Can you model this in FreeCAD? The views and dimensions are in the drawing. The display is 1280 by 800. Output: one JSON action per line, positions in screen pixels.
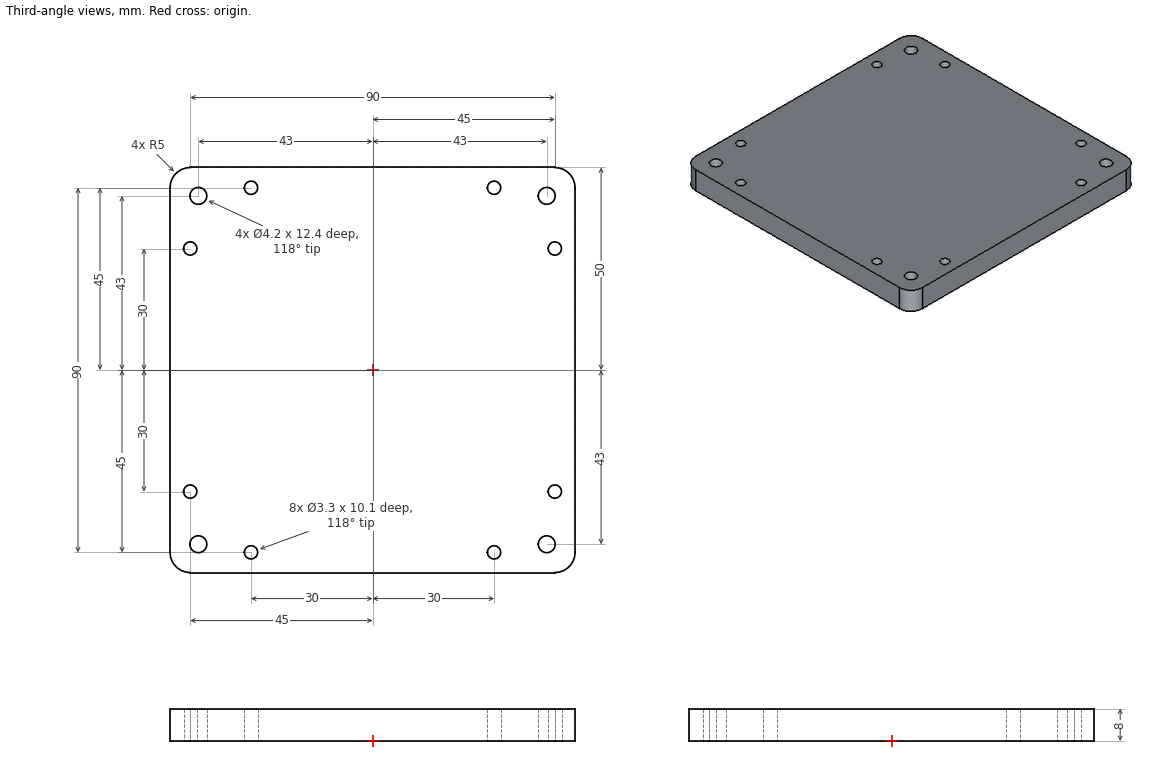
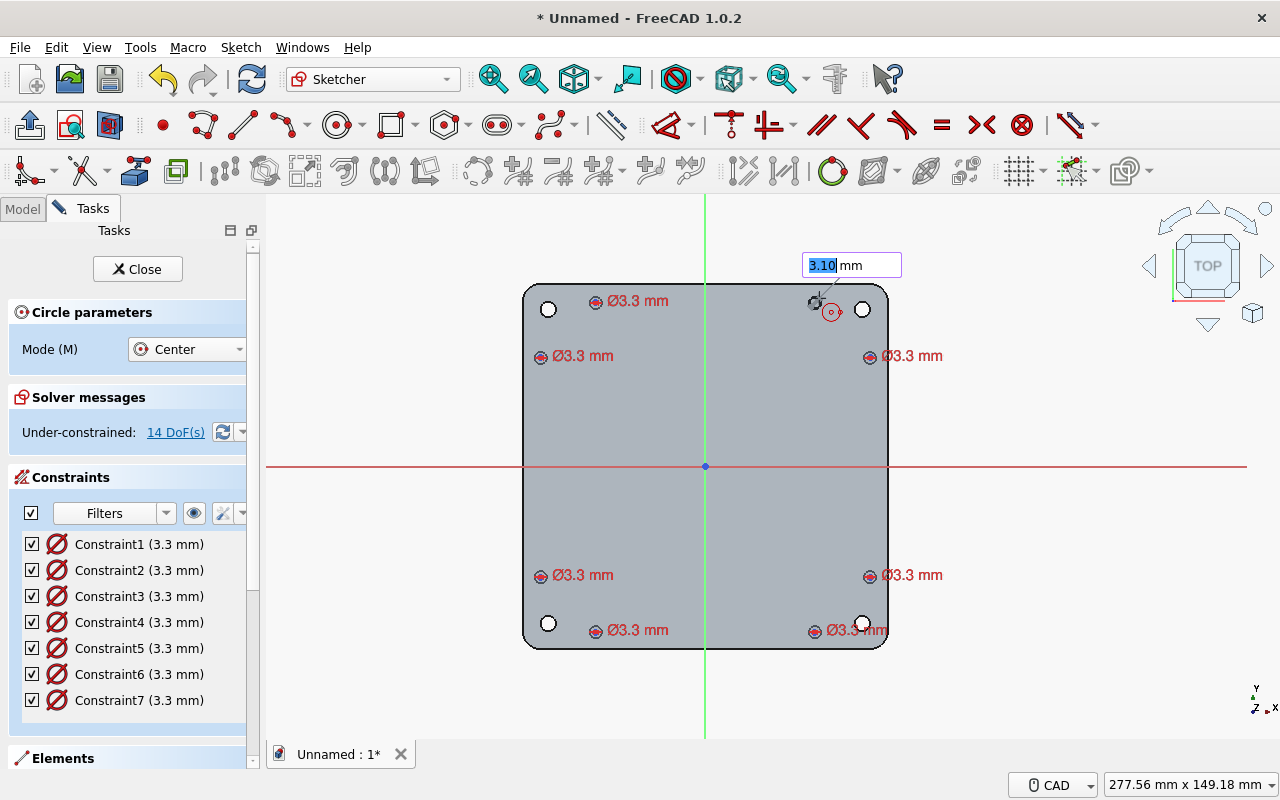
{"action": "type", "text": "3.3"}
{"action": "key", "text": "Return"}
{"action": "key", "text": "Escape"}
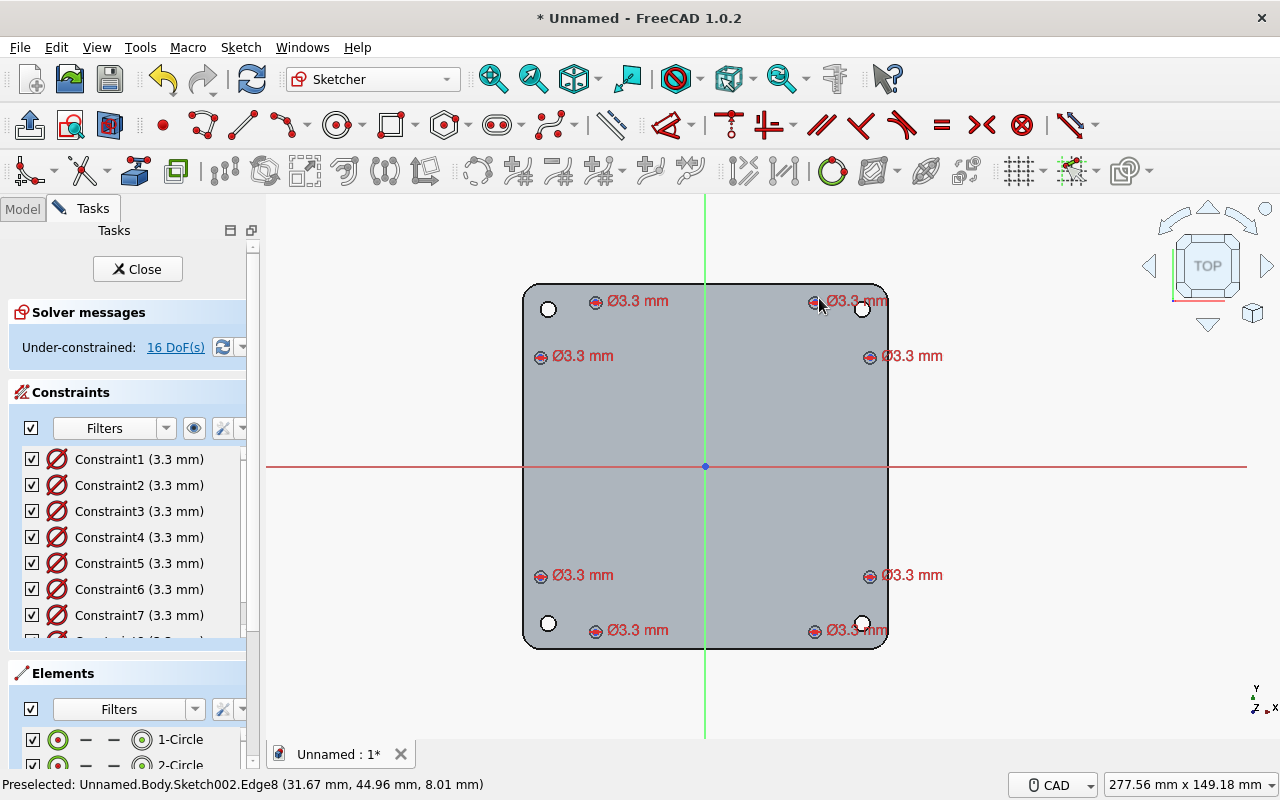
{"action": "left_click", "coordinate": [596, 632]}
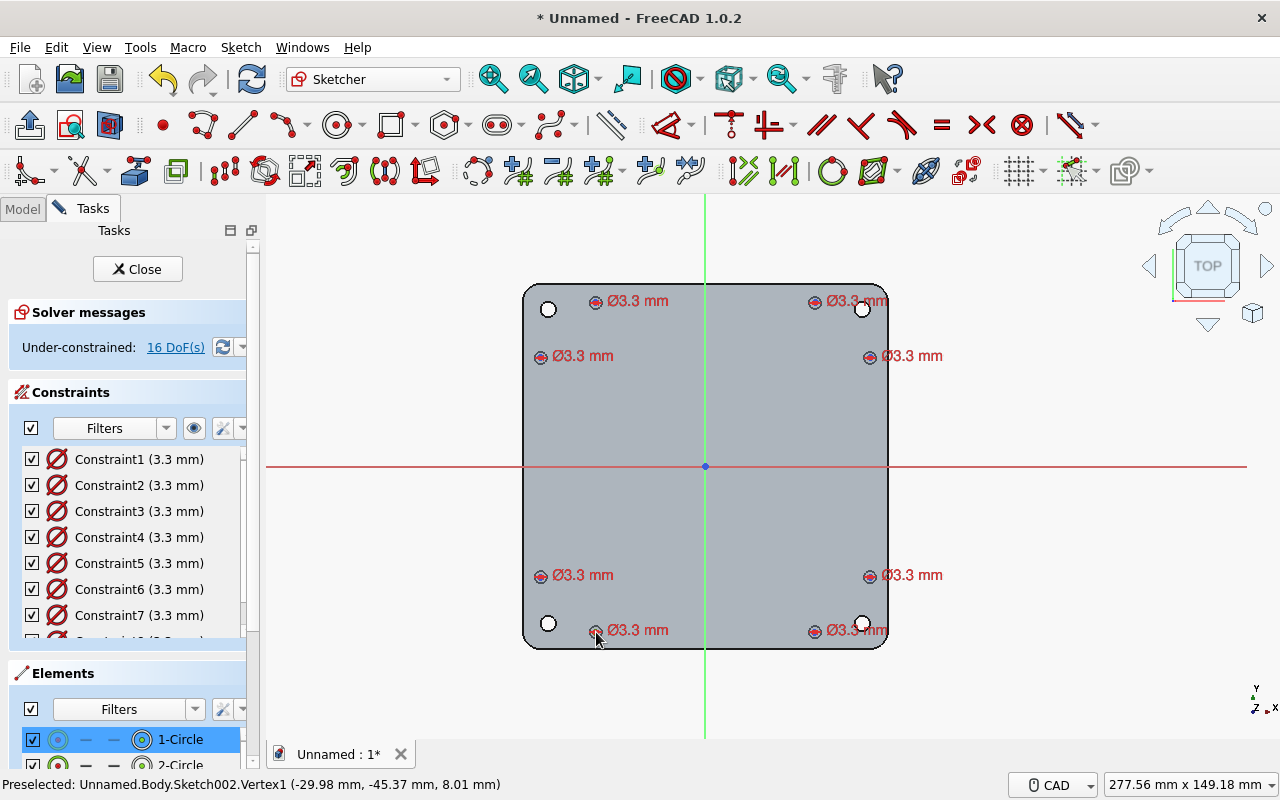
{"action": "left_click", "coordinate": [815, 632]}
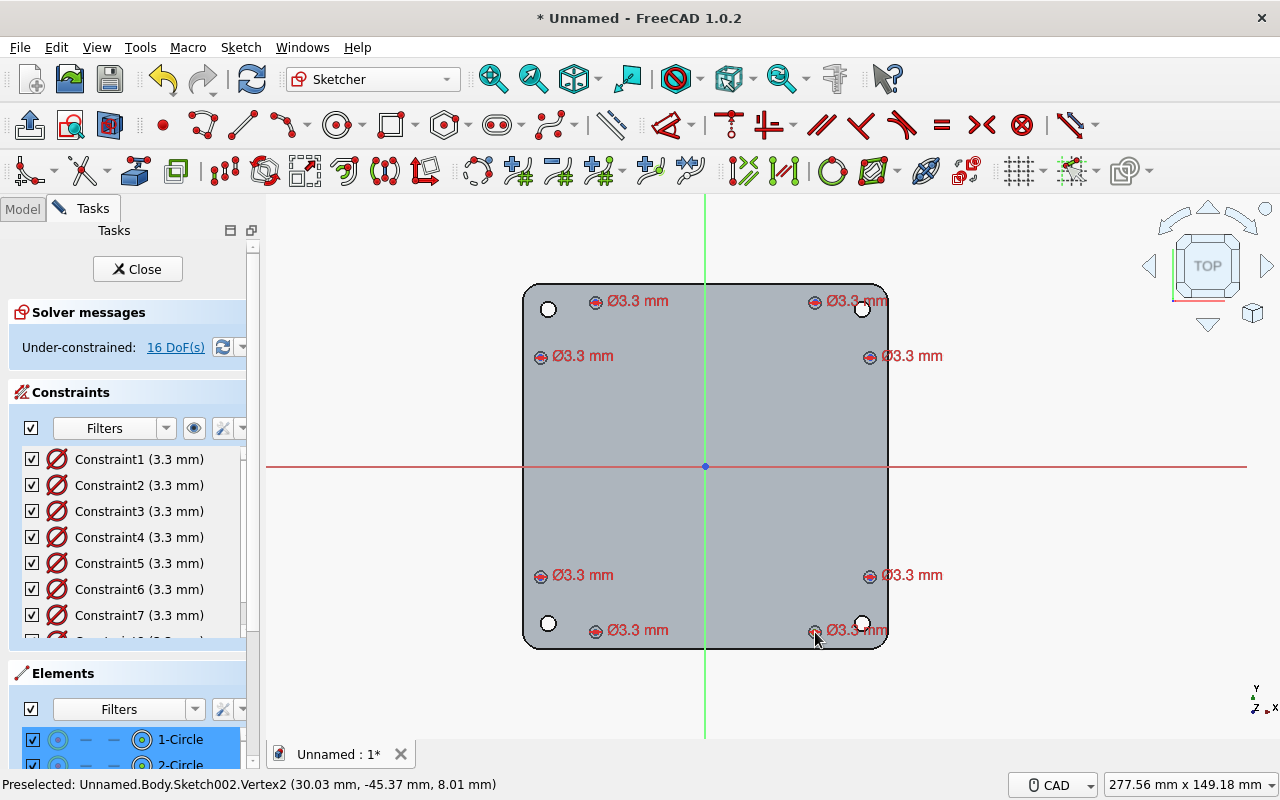
{"action": "key", "text": "h"}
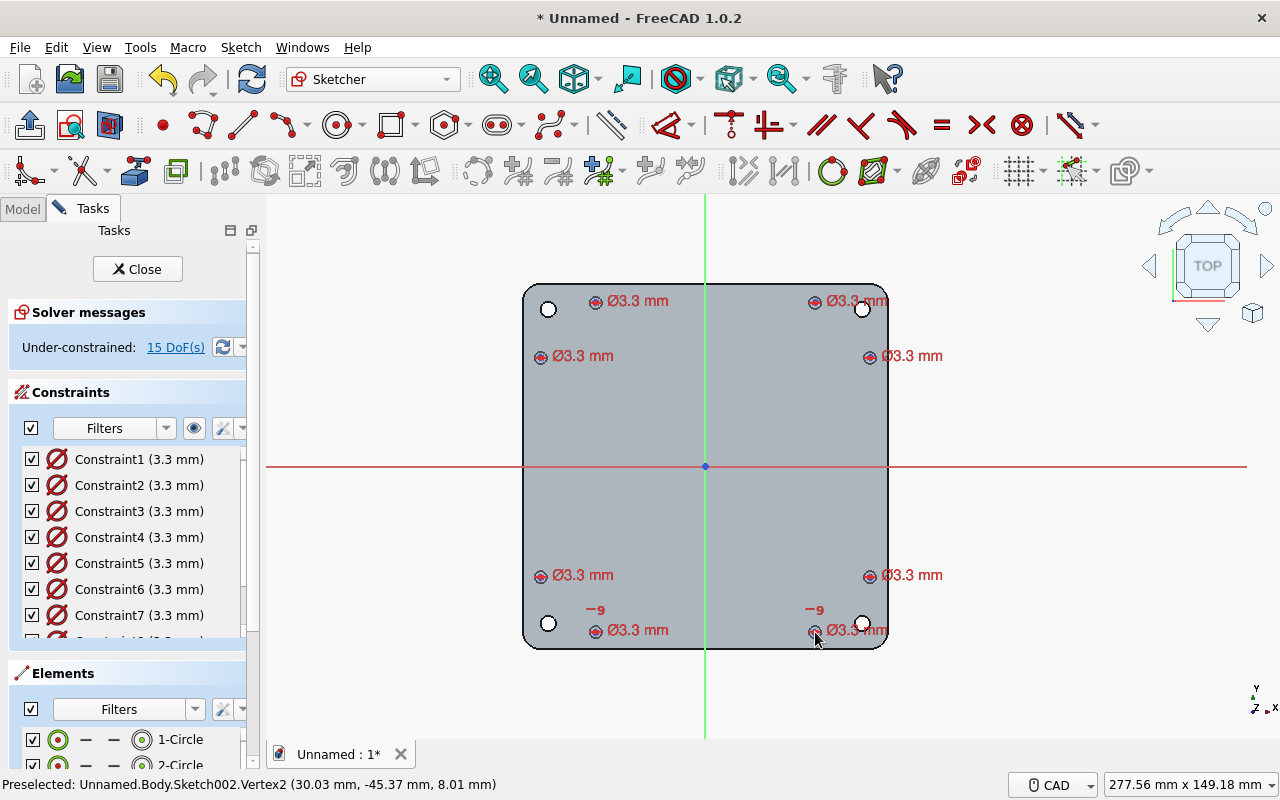
{"action": "left_click", "coordinate": [541, 577]}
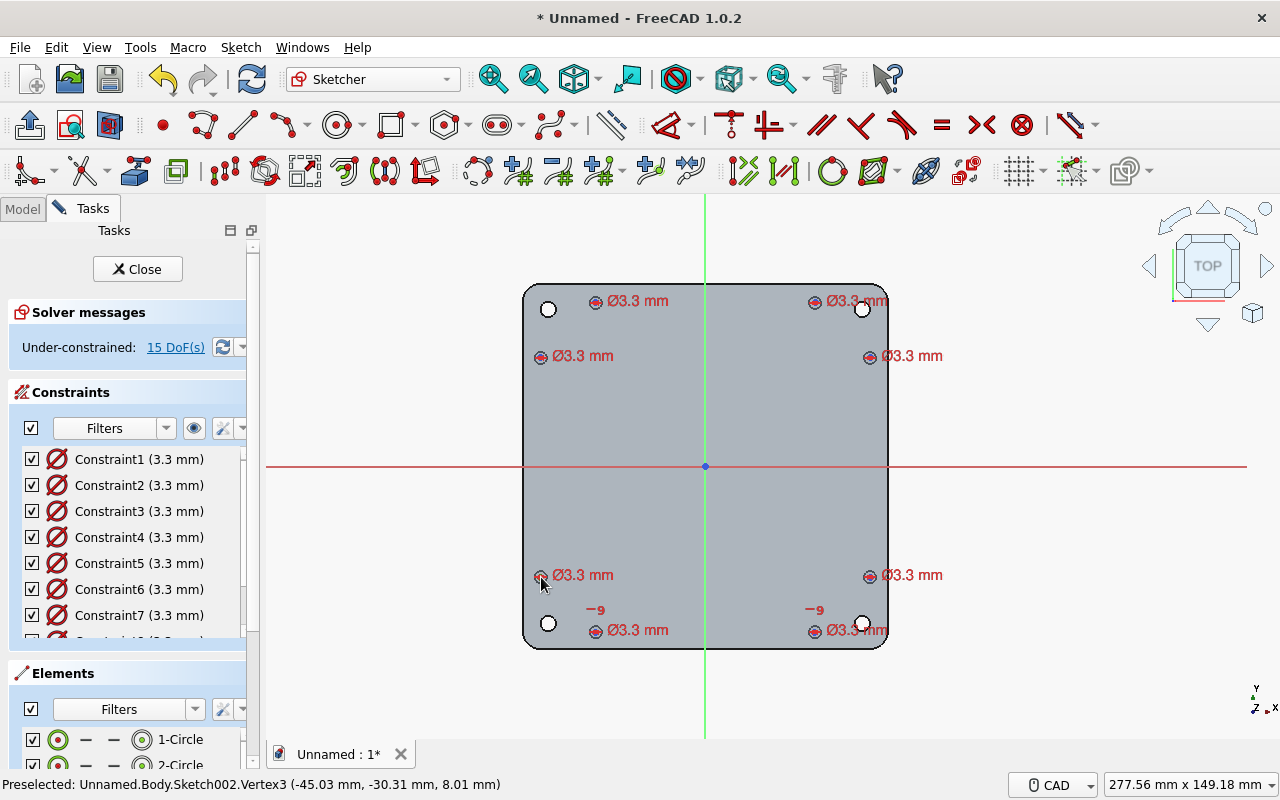
{"action": "left_click", "coordinate": [541, 358]}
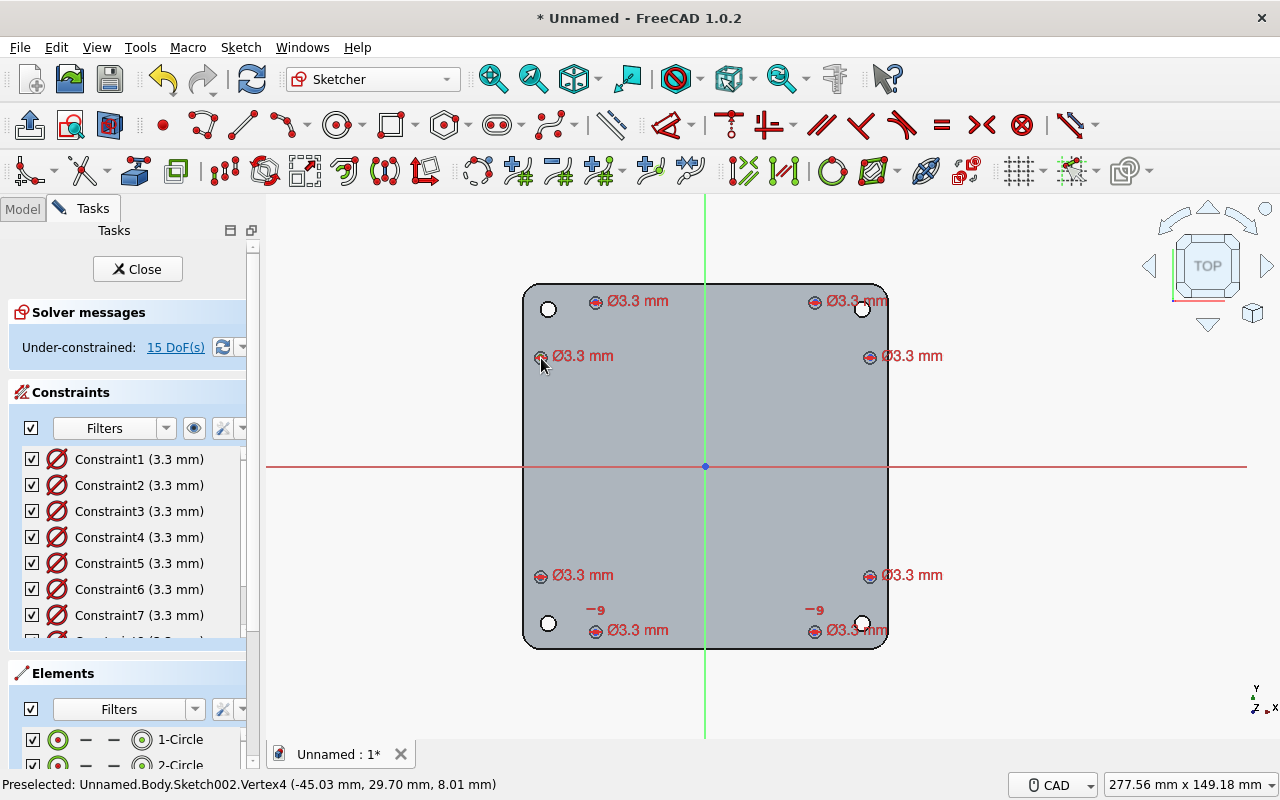
{"action": "key", "text": "v"}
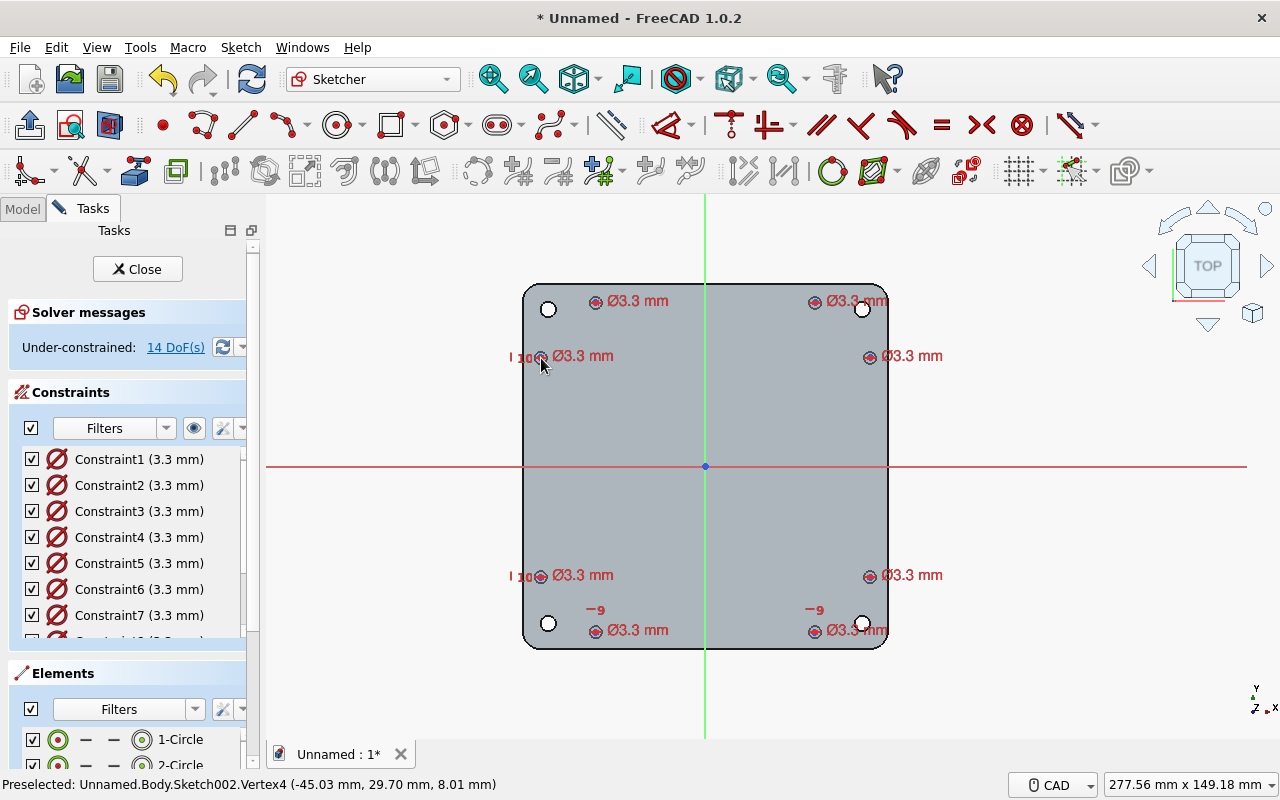
{"action": "left_click", "coordinate": [541, 358]}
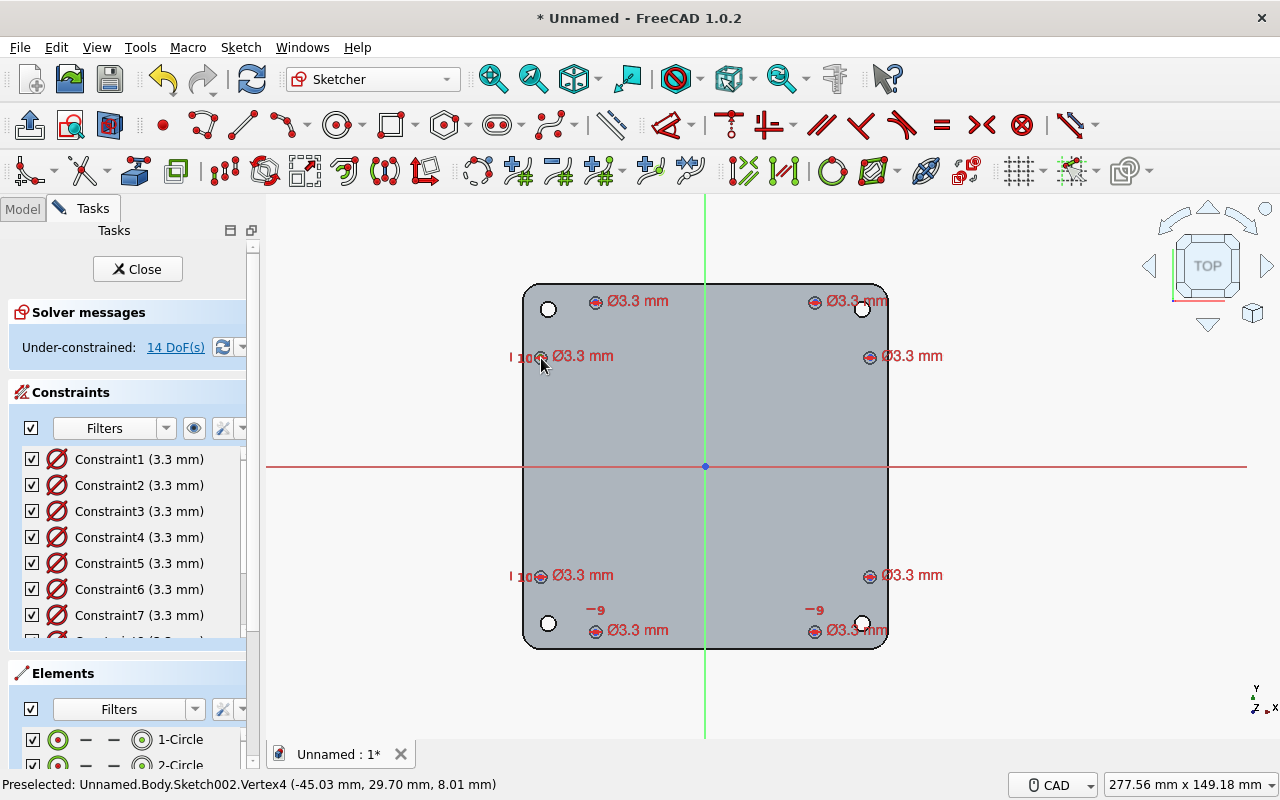
{"action": "left_click", "coordinate": [870, 358]}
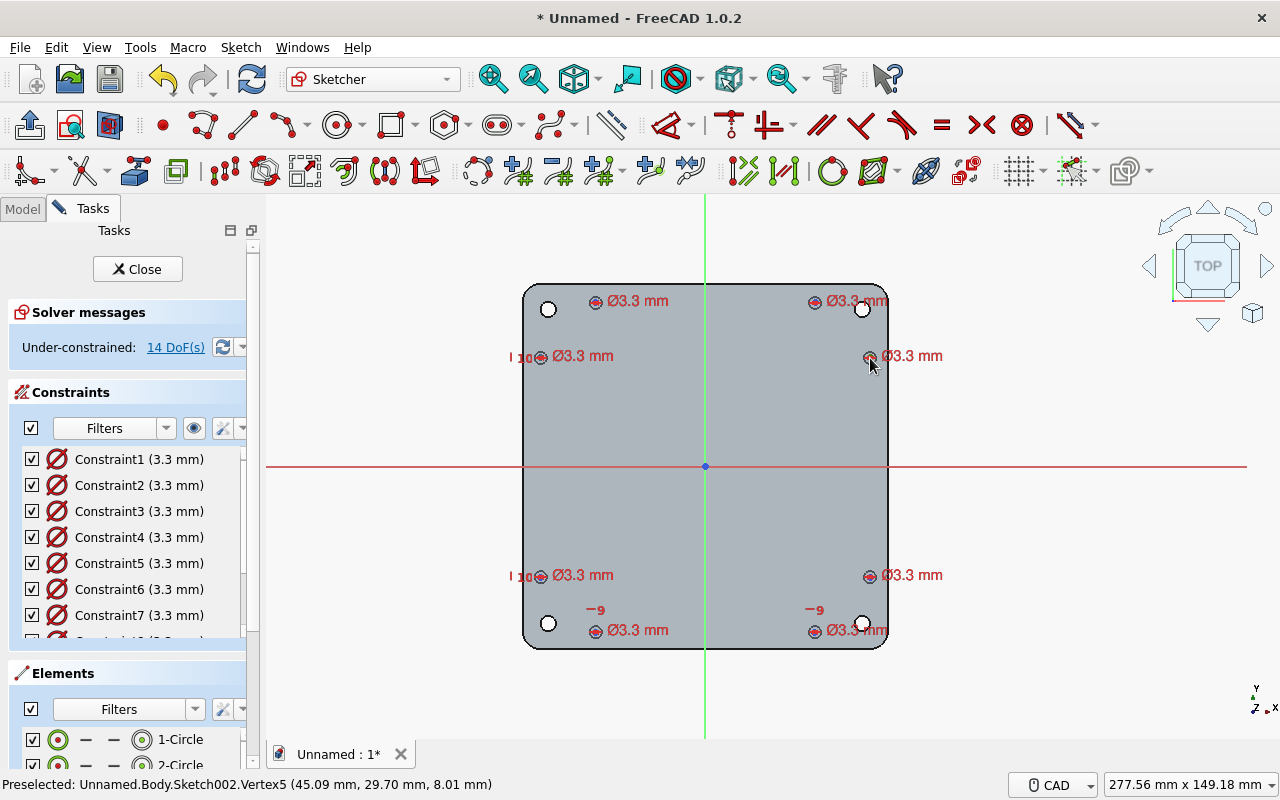
{"action": "key", "text": "h"}